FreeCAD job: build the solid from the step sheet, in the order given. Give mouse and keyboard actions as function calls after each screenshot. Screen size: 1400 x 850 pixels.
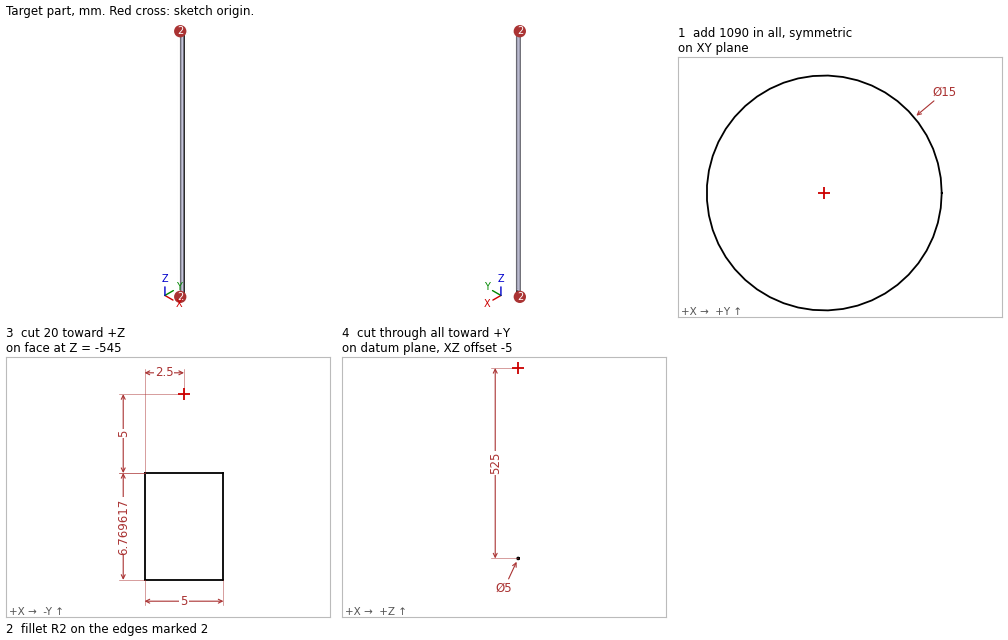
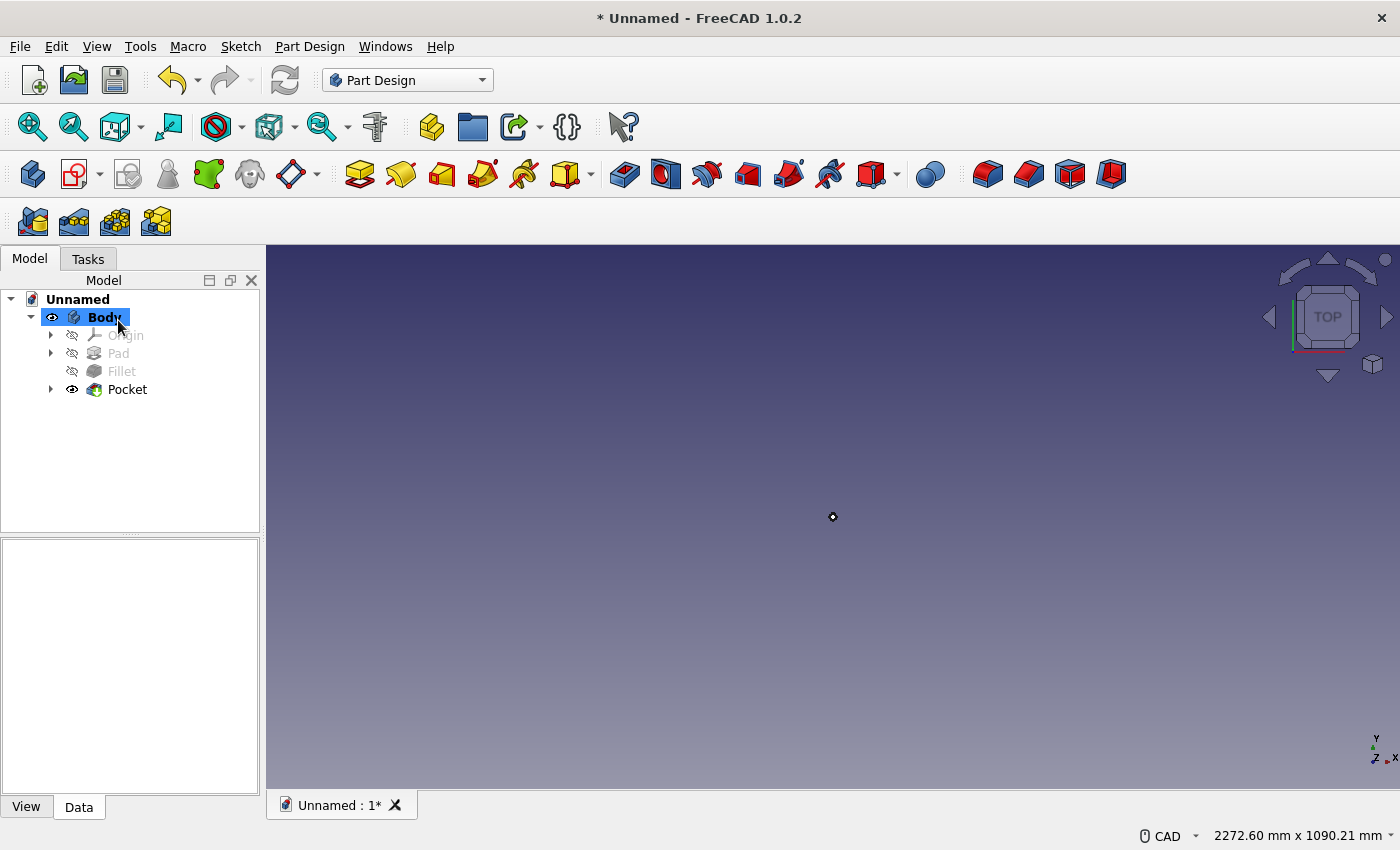
key(v)
key(f)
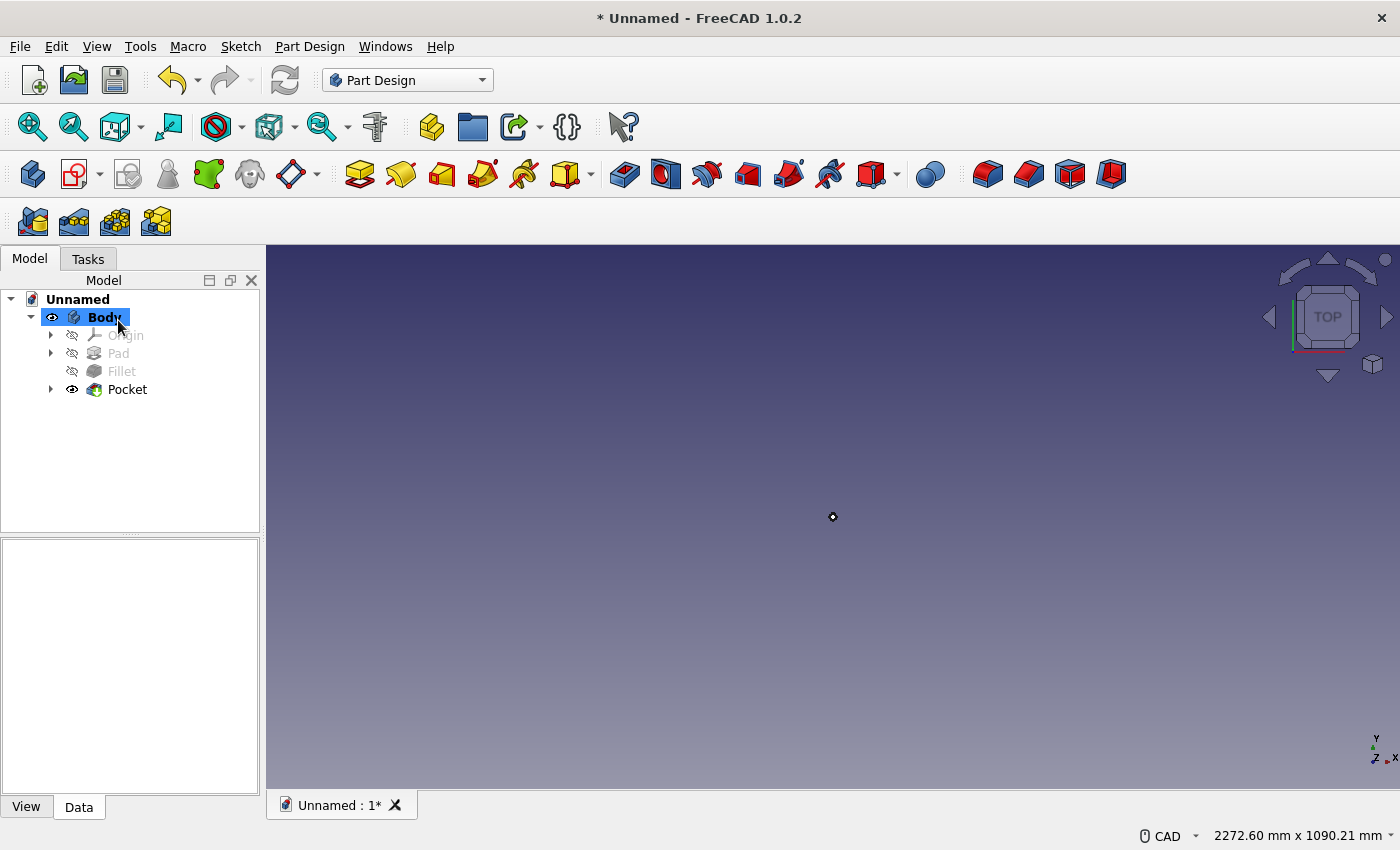
key(3)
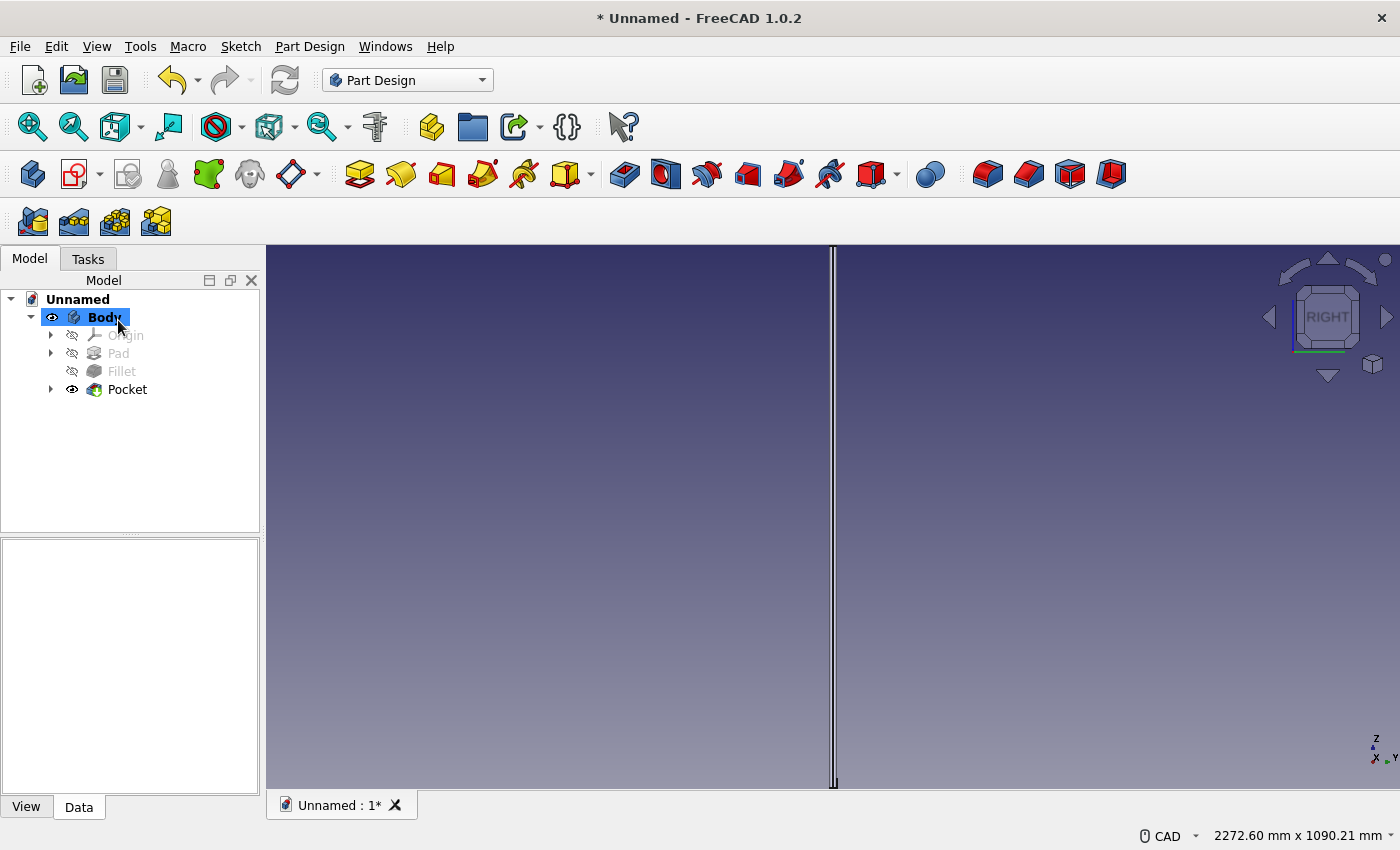
key(v)
key(f)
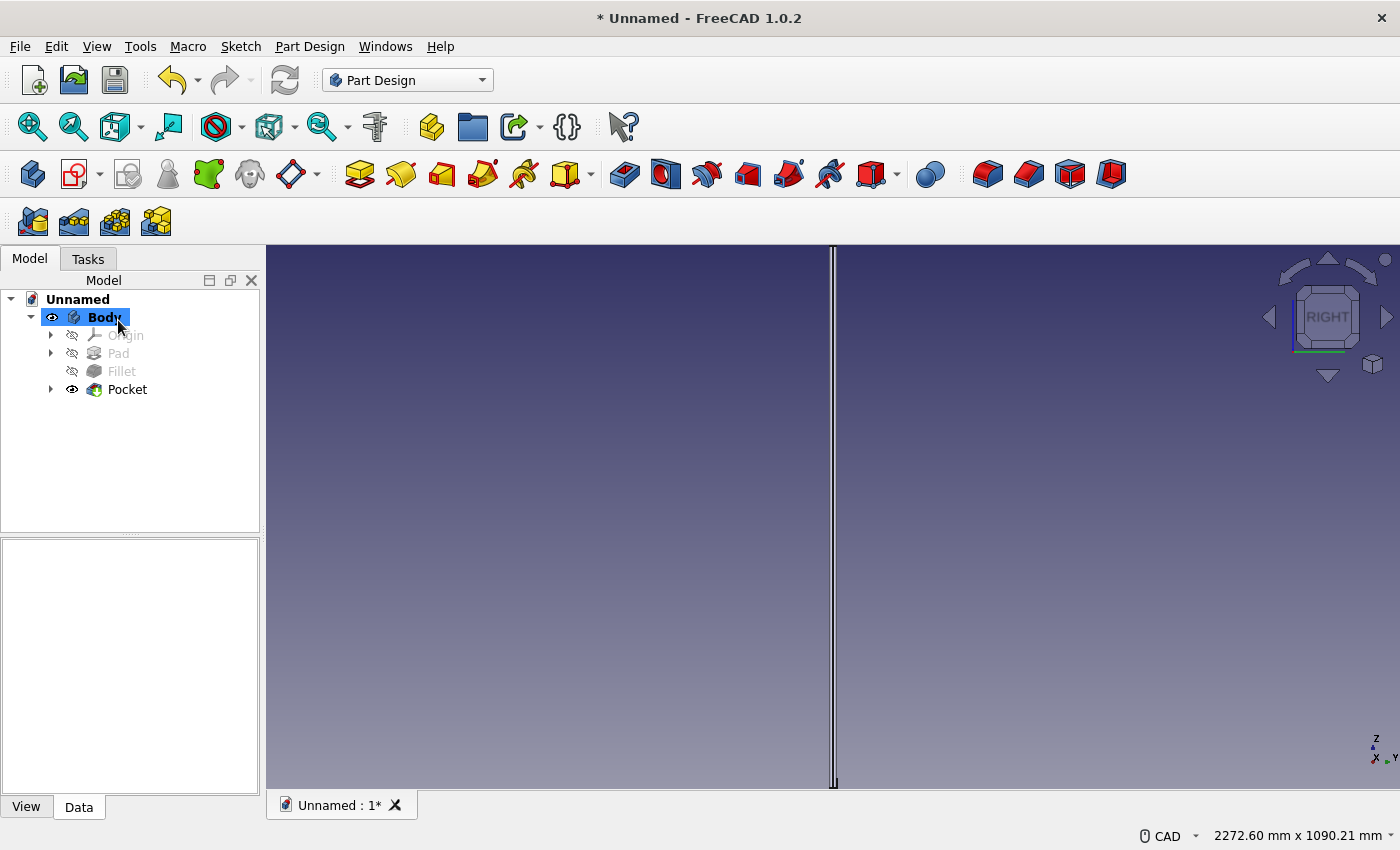
click(51, 335)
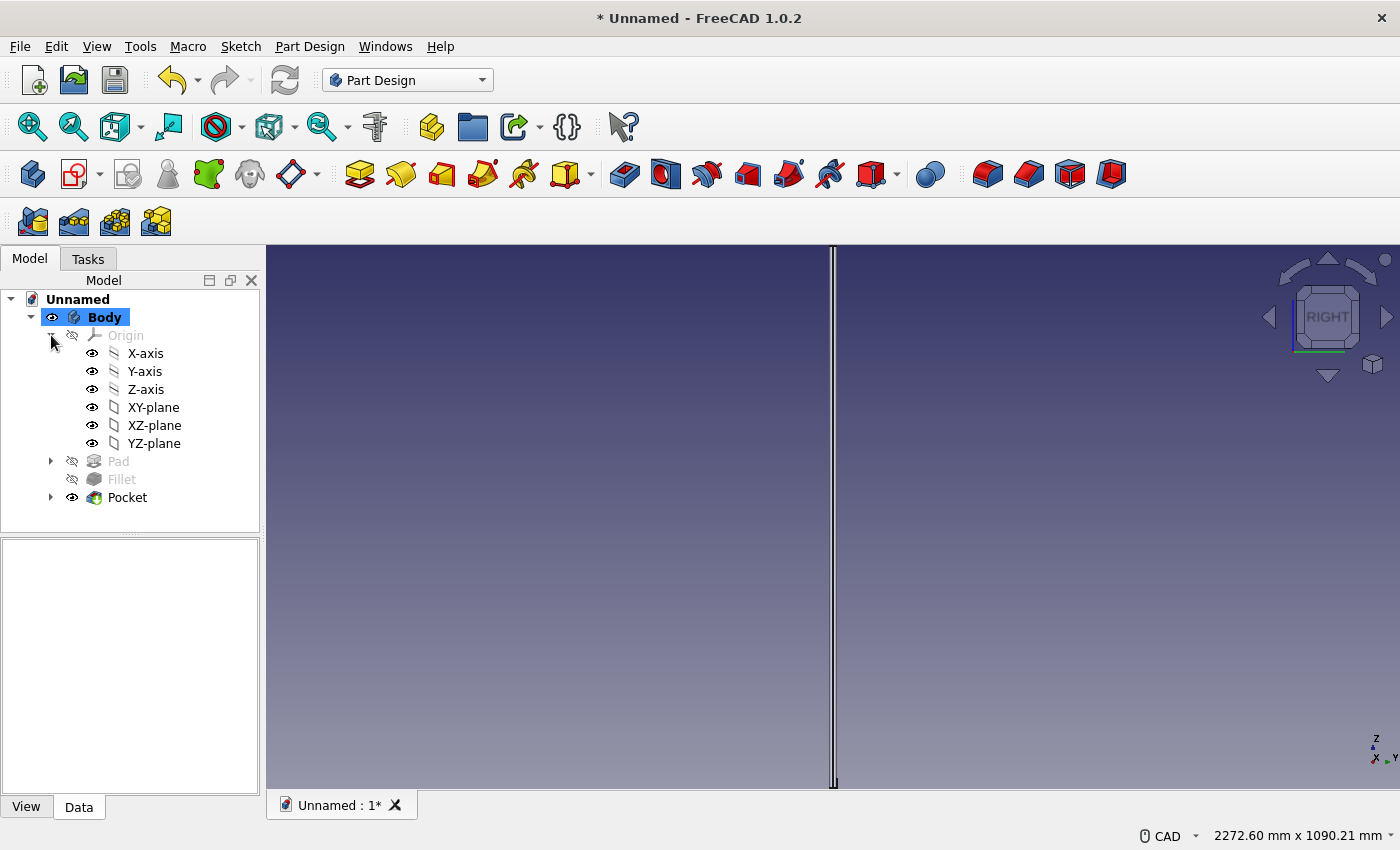
click(137, 425)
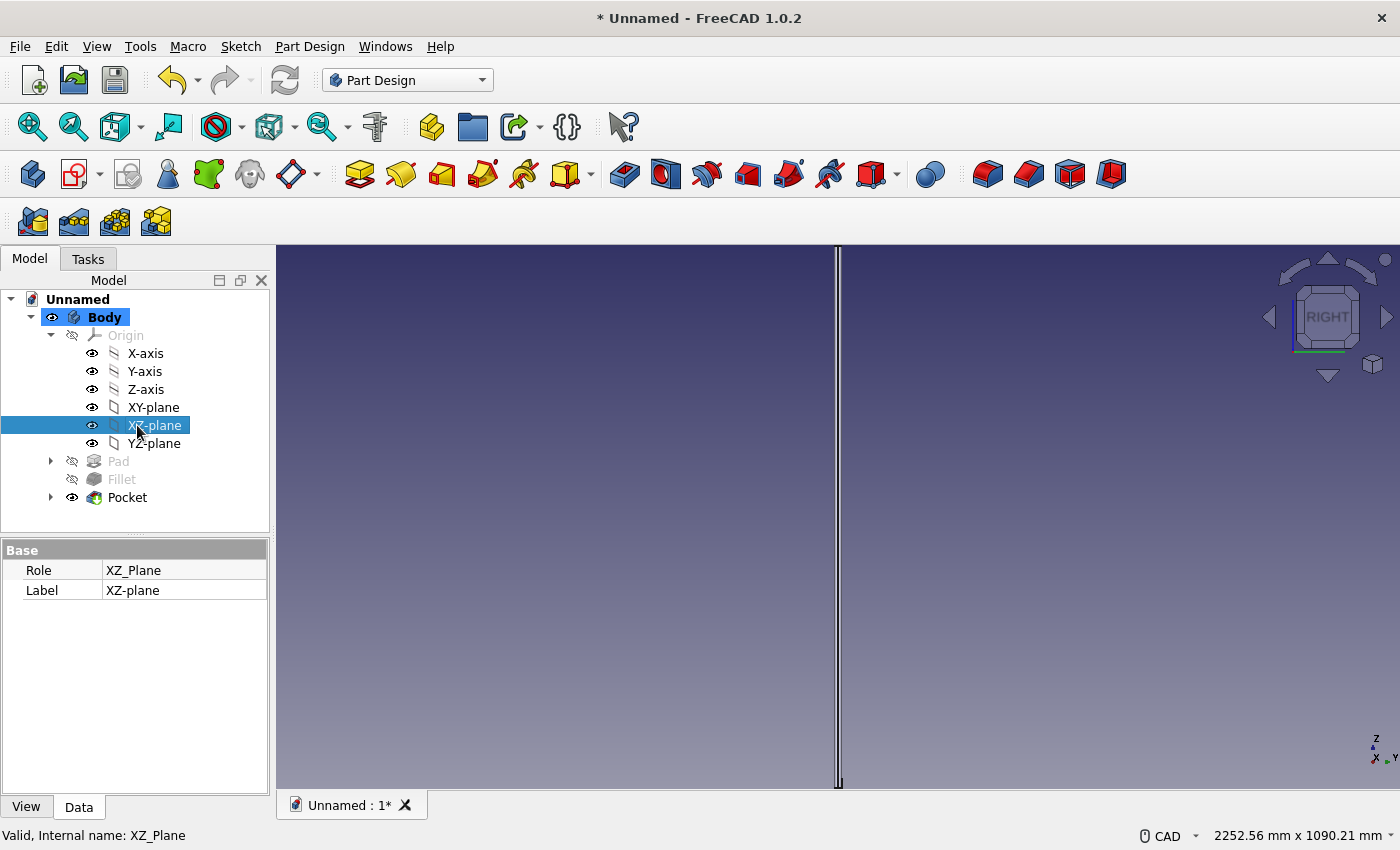
click(290, 174)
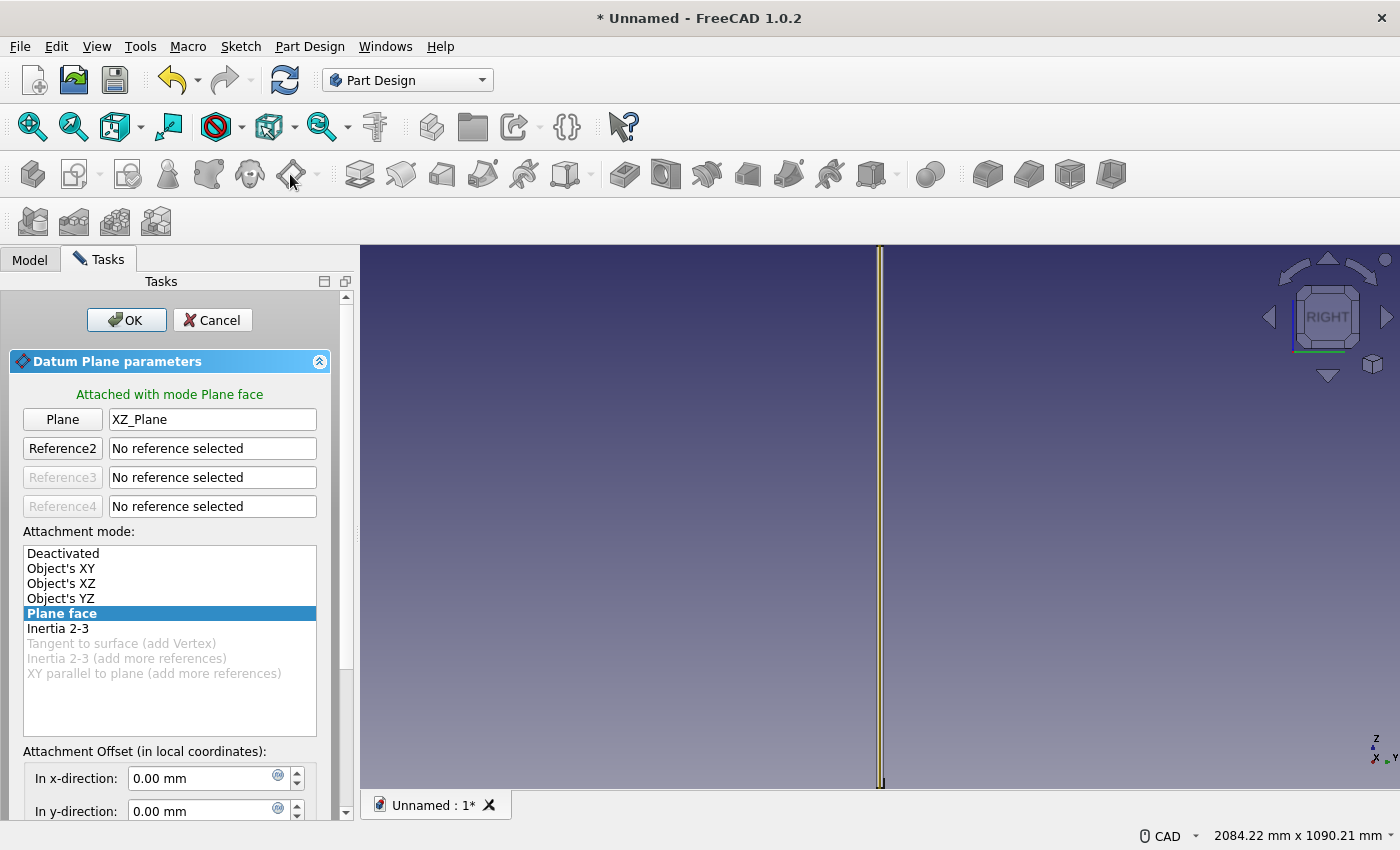
scroll(346, 556, down, 2)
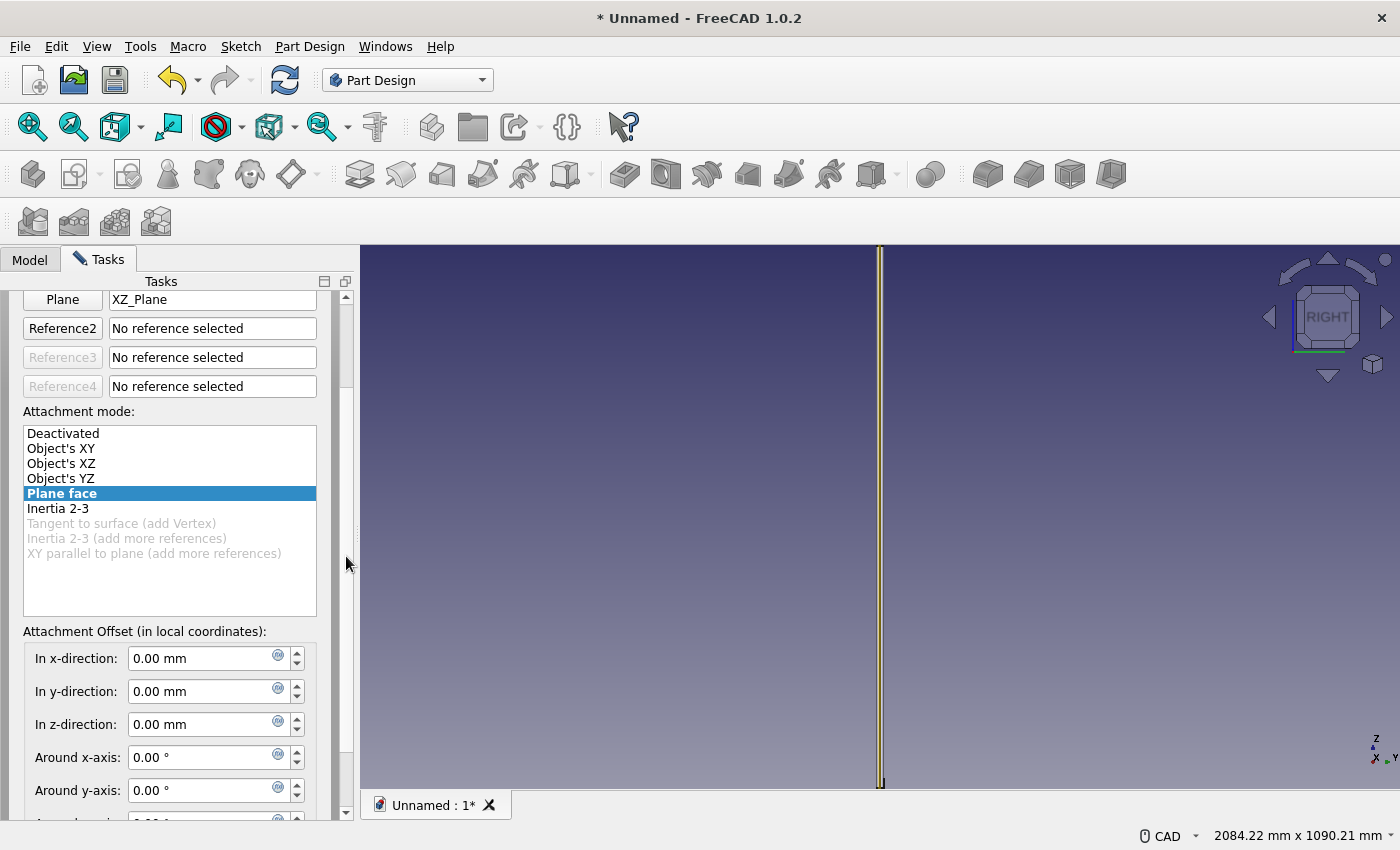
triple_click(210, 724)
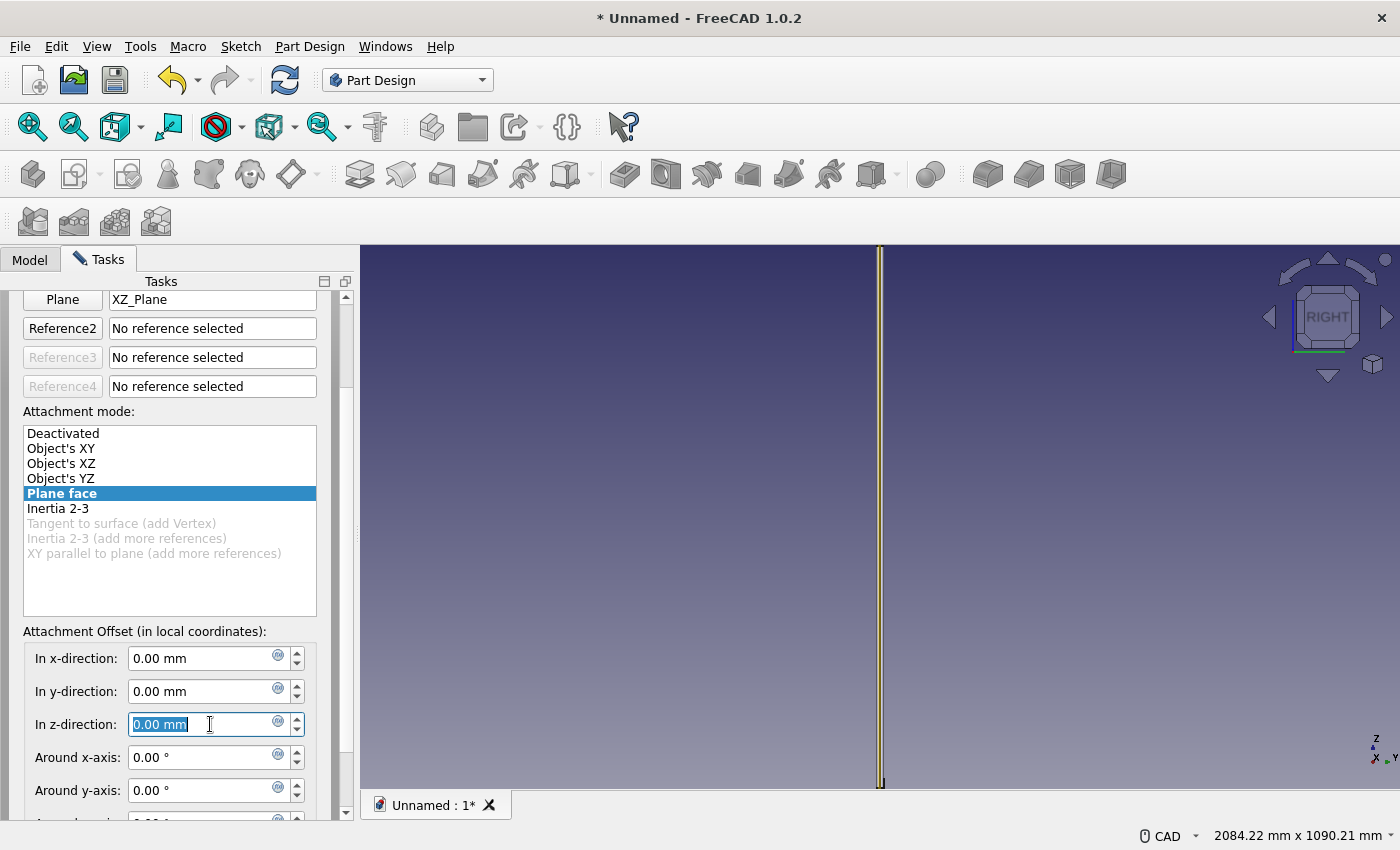
text(-5)
key(Tab)